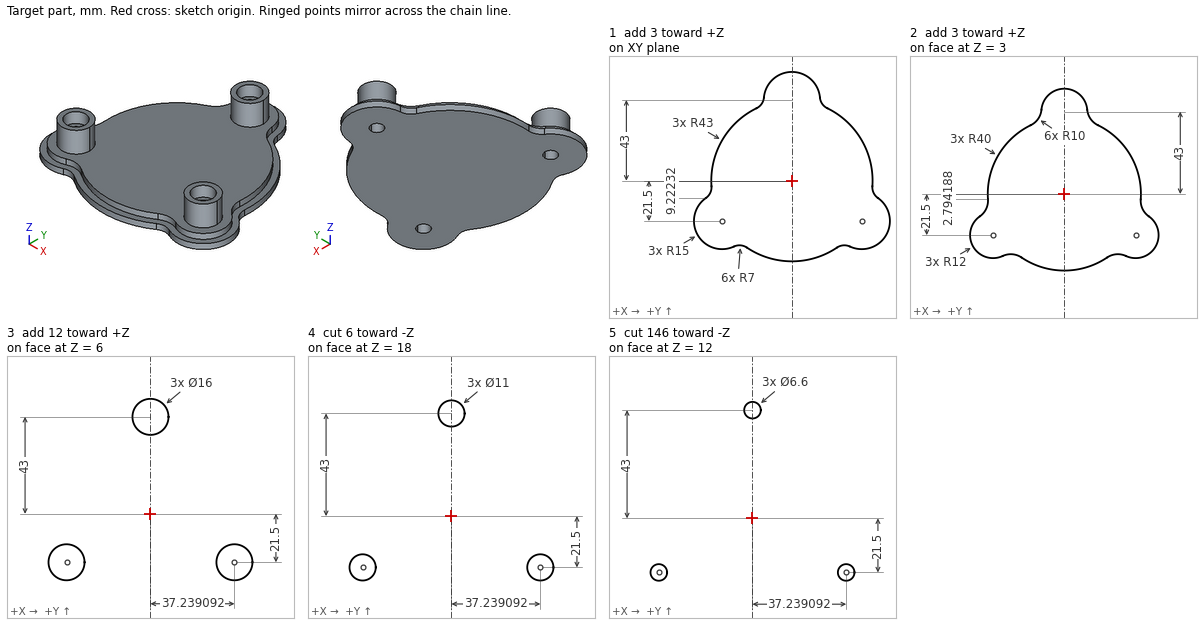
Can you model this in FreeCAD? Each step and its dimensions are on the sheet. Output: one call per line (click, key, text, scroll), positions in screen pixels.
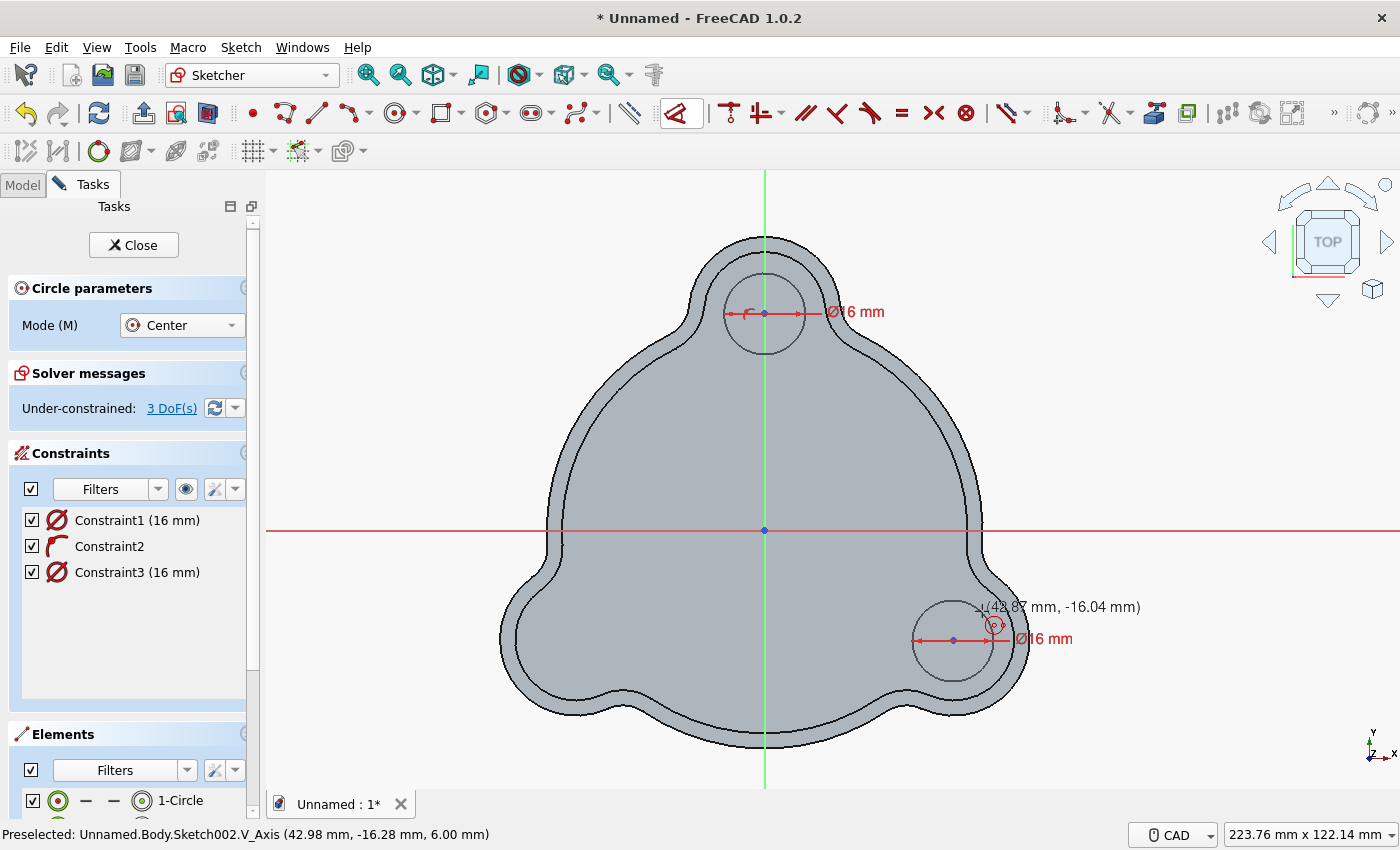
click(576, 640)
move(605, 611)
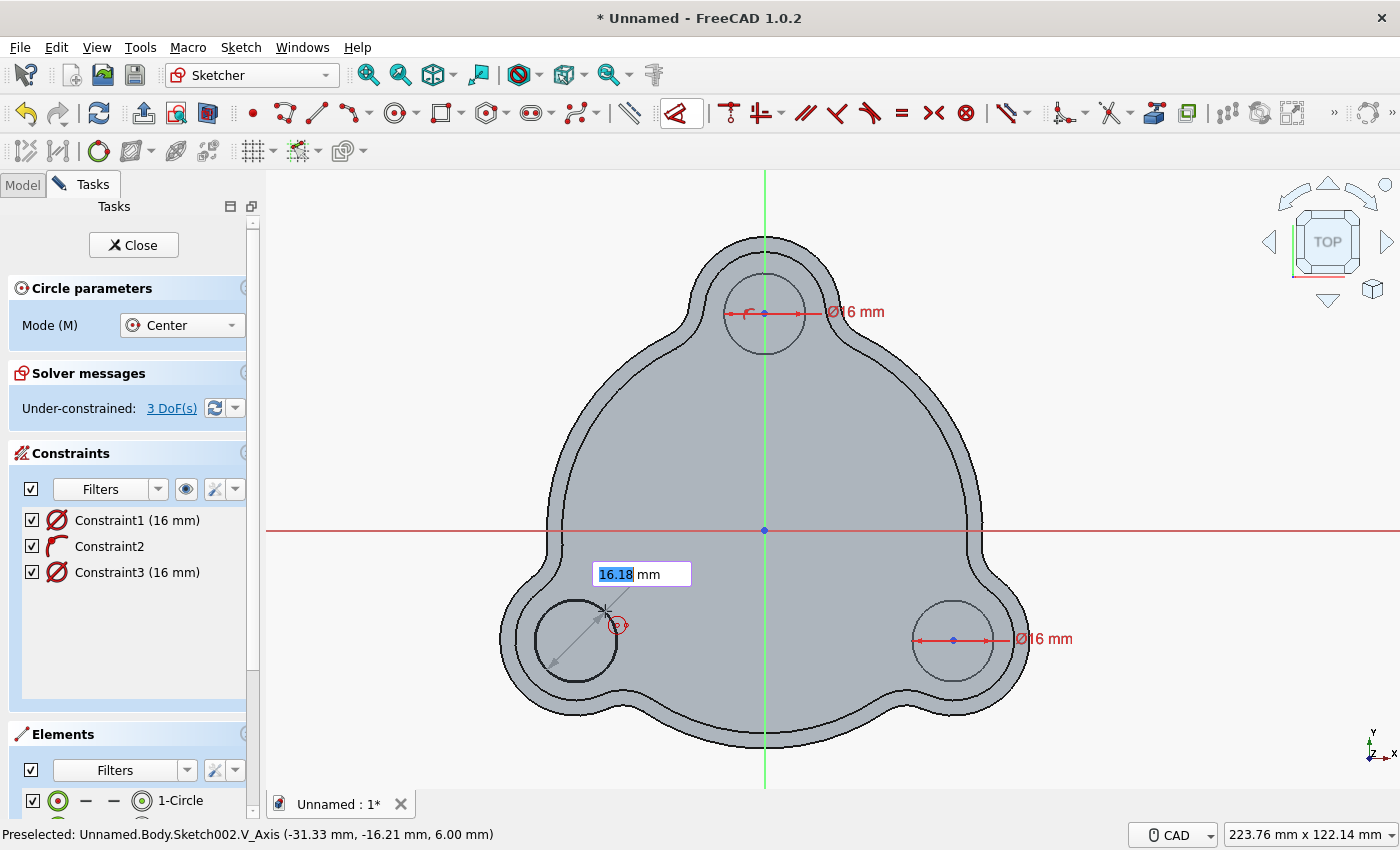
text(16)
key(Return)
key(Escape)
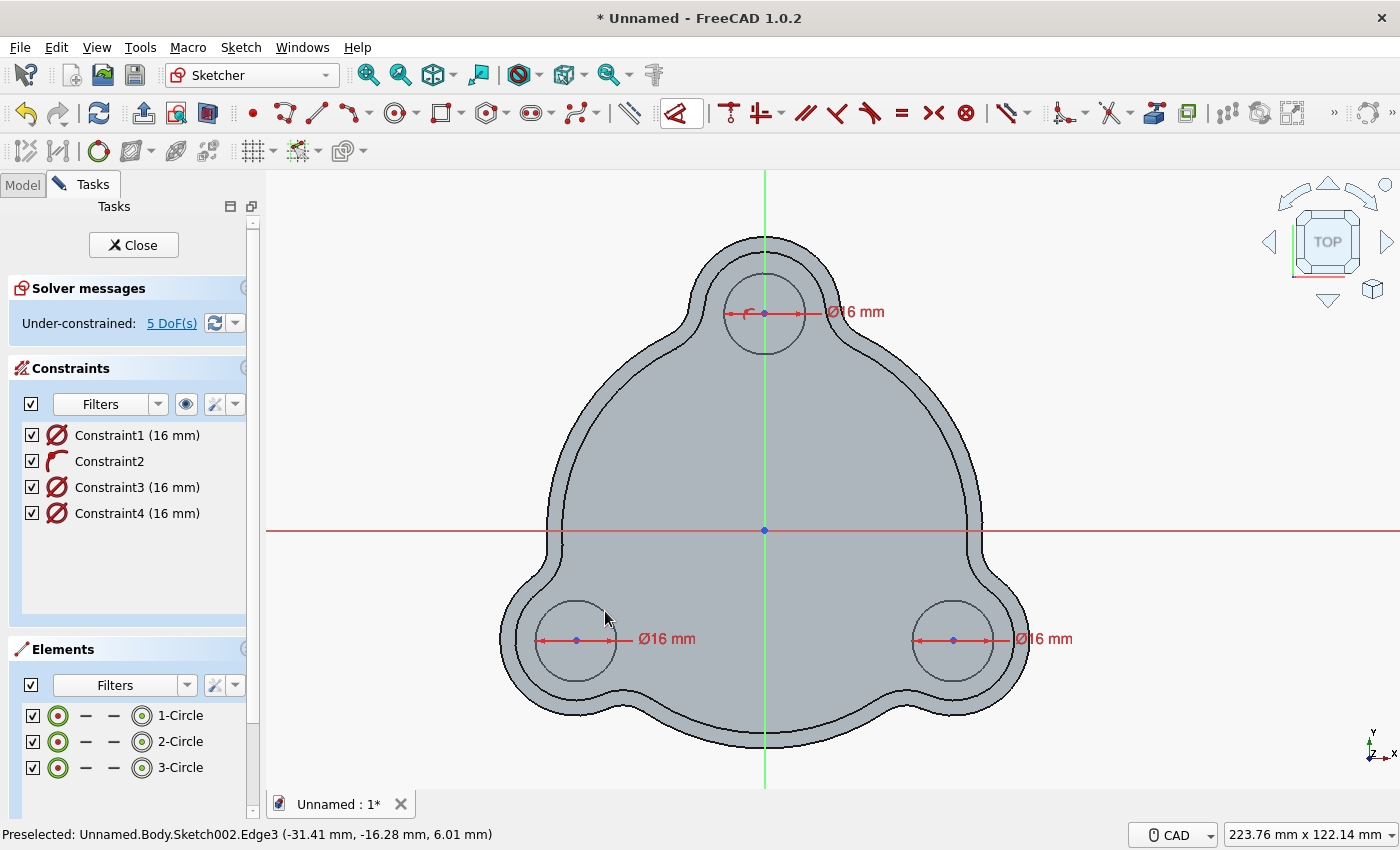
click(953, 641)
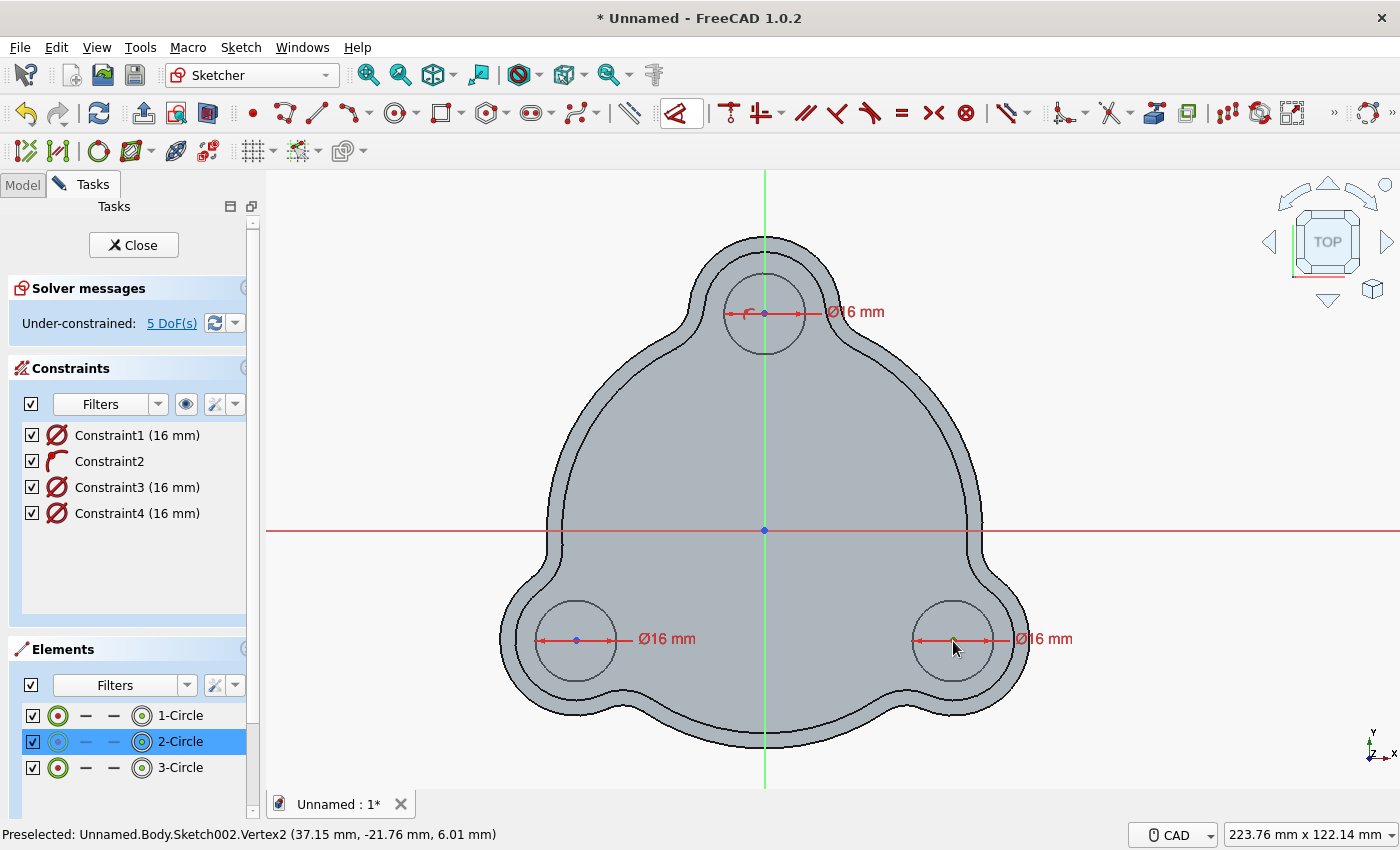
click(576, 641)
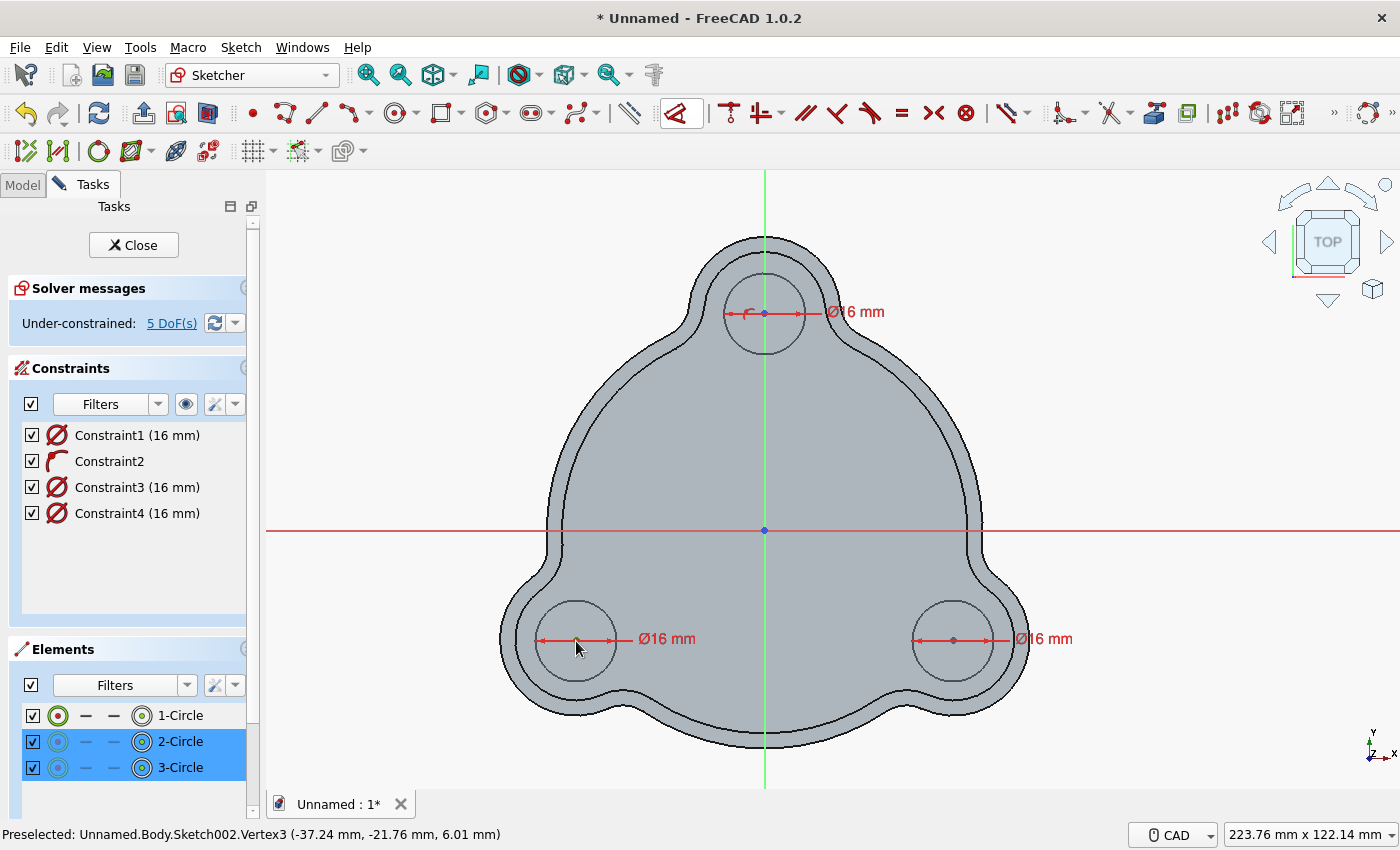
click(765, 721)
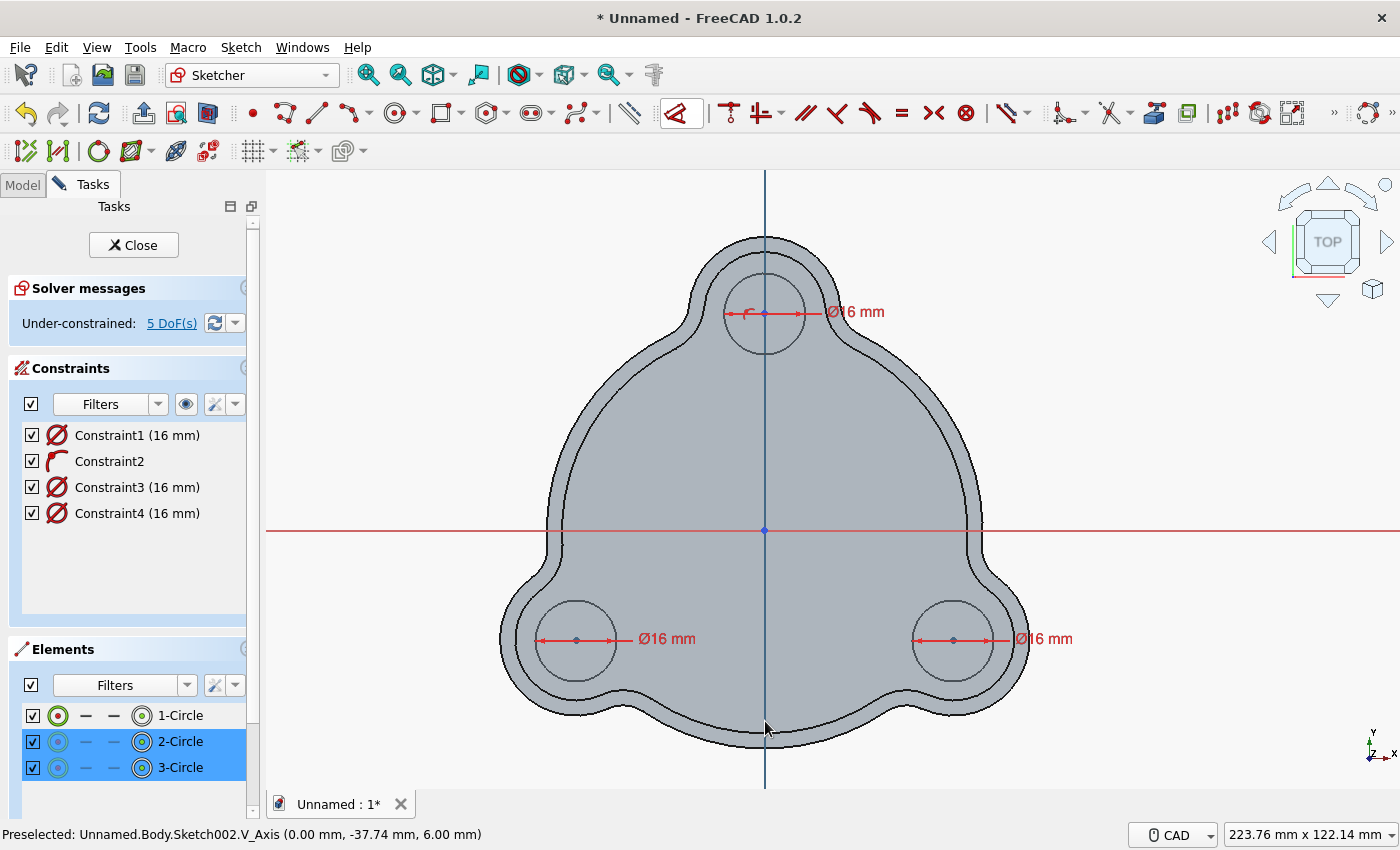
key(s)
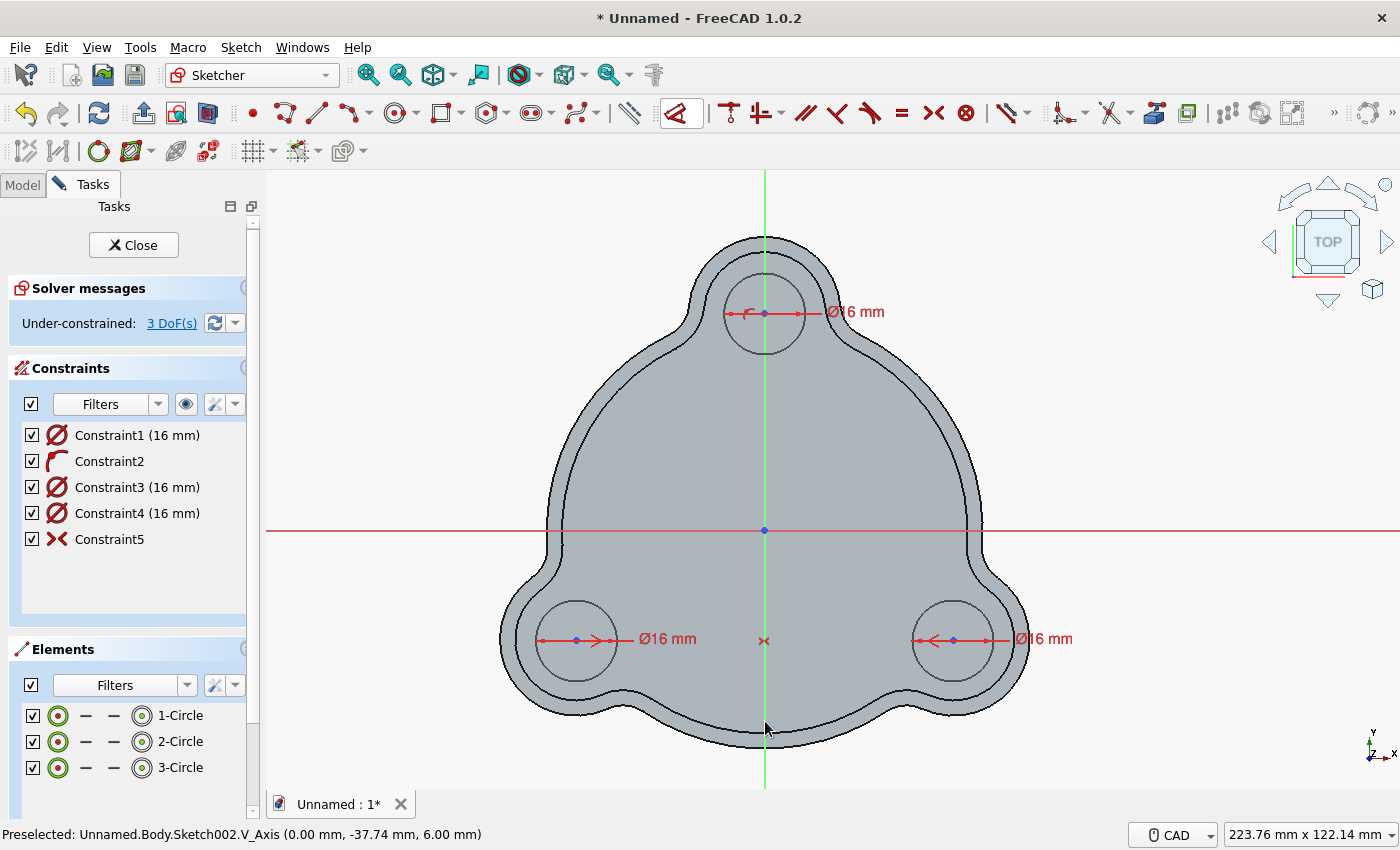
click(765, 314)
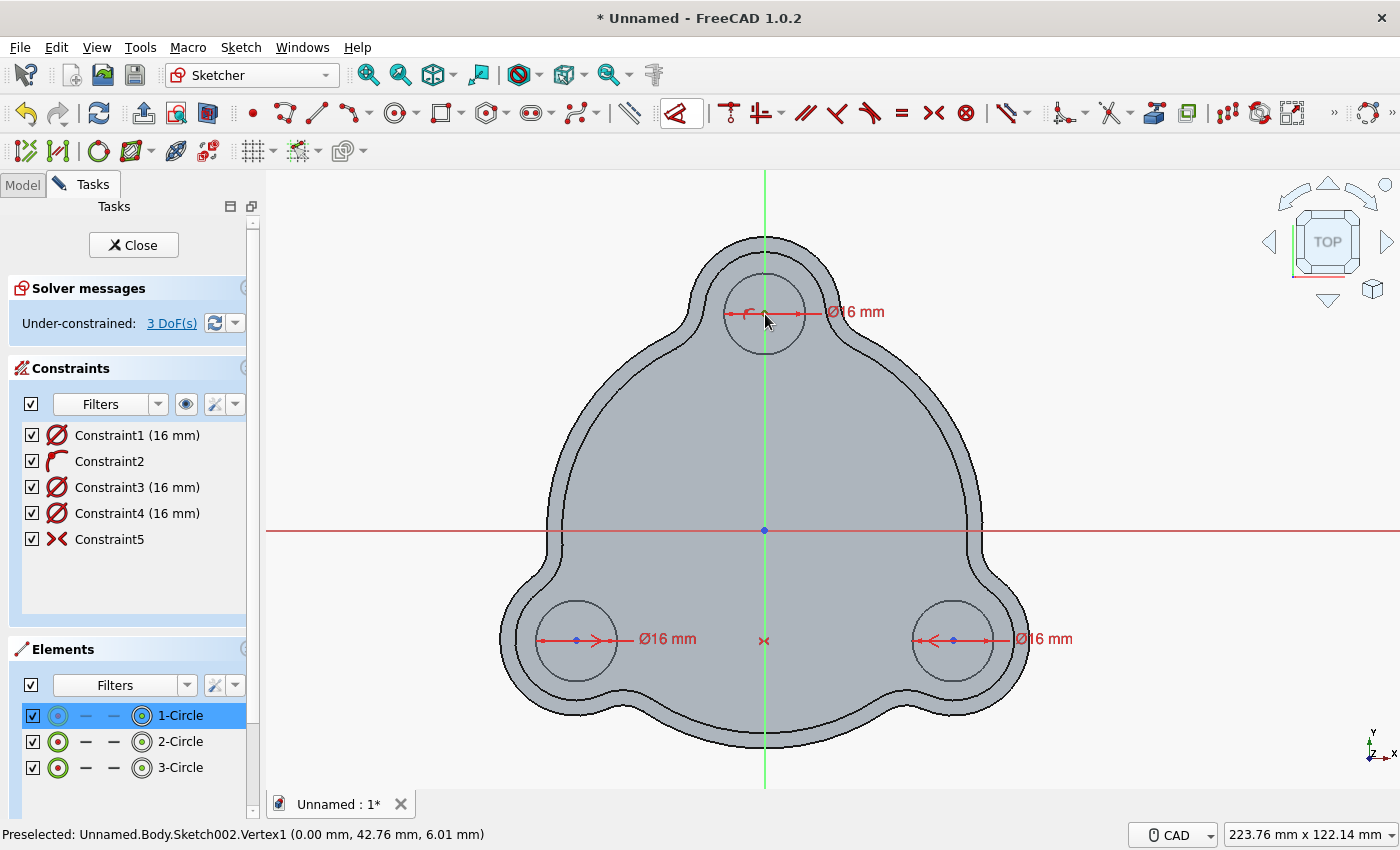
click(698, 114)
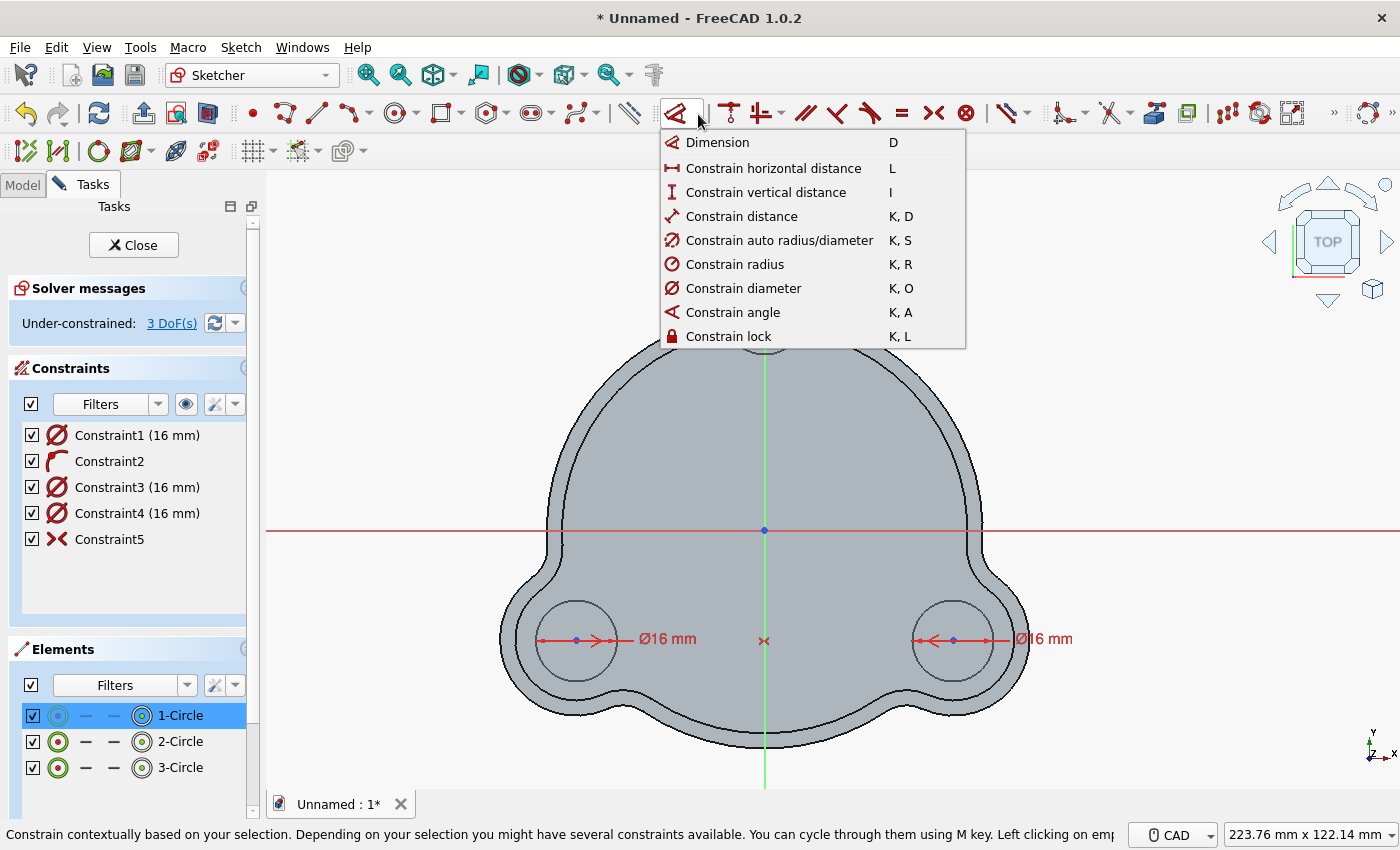
click(813, 192)